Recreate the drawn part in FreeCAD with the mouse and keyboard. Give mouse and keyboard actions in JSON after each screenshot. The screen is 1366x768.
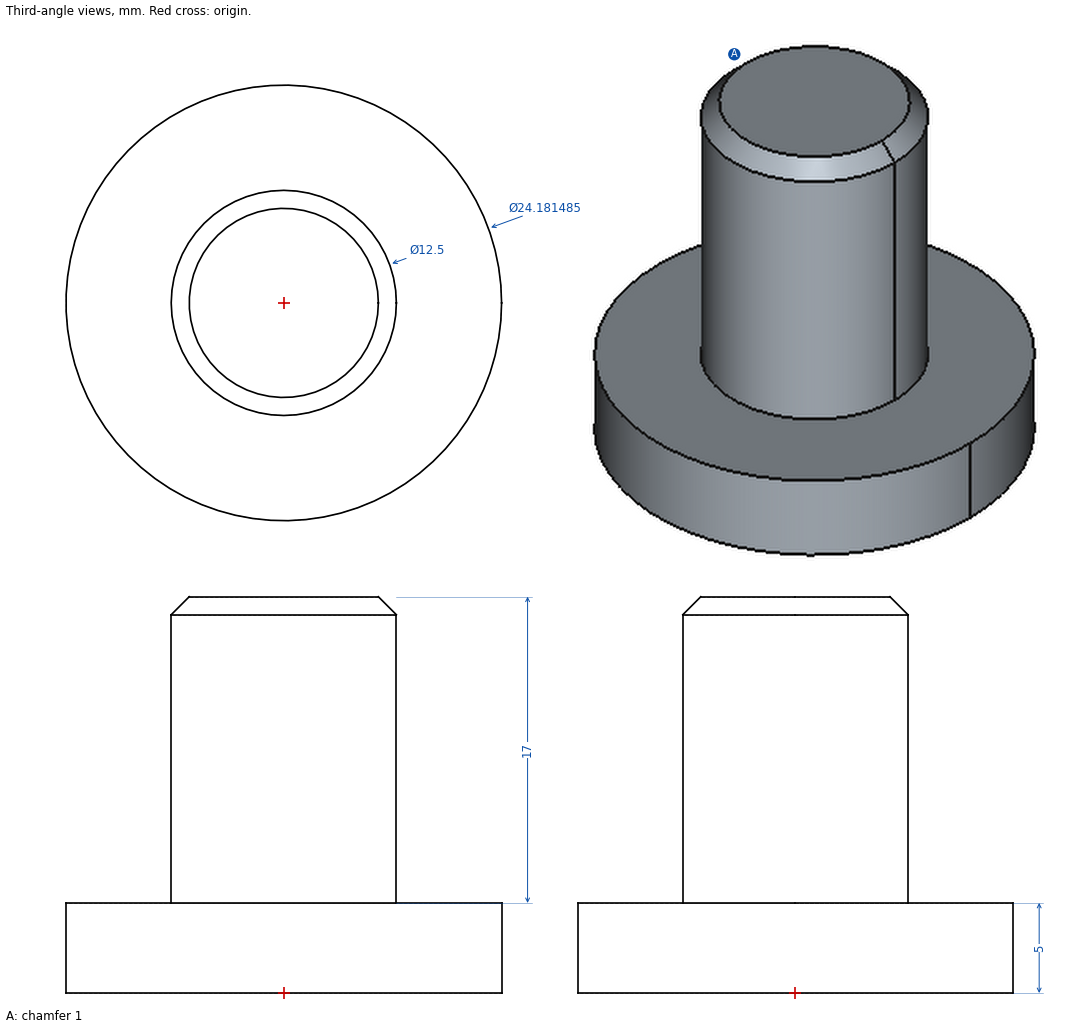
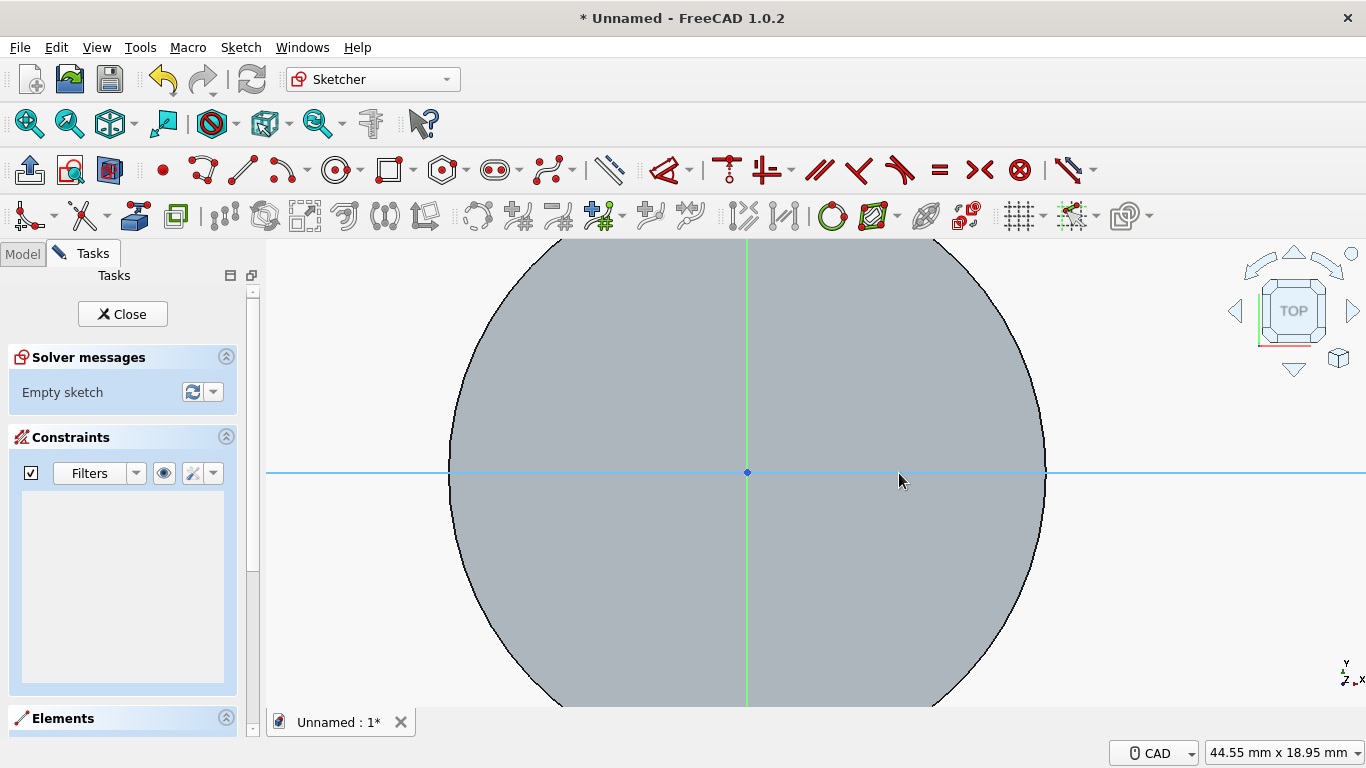
{"action": "left_click", "coordinate": [336, 170]}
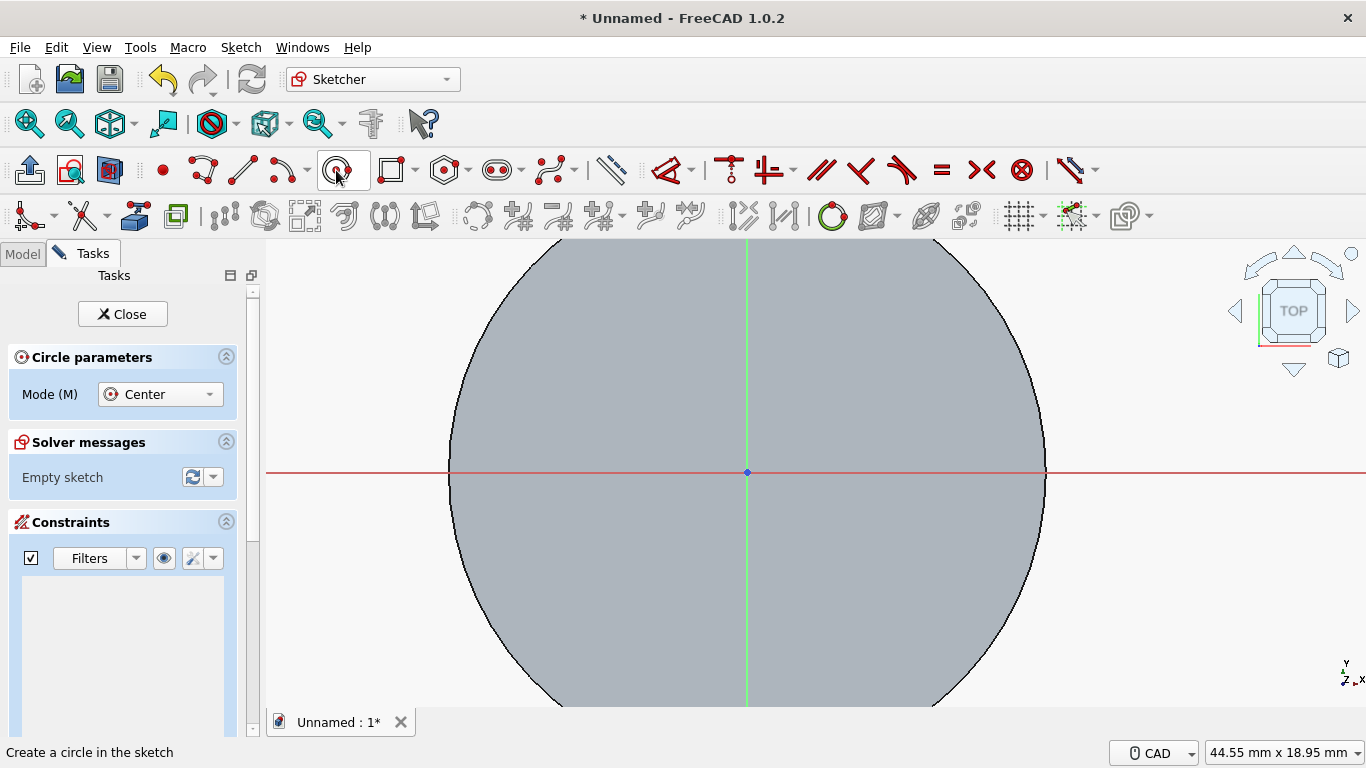
{"action": "left_click", "coordinate": [747, 473]}
{"action": "left_click", "coordinate": [856, 363]}
{"action": "key", "text": "Escape"}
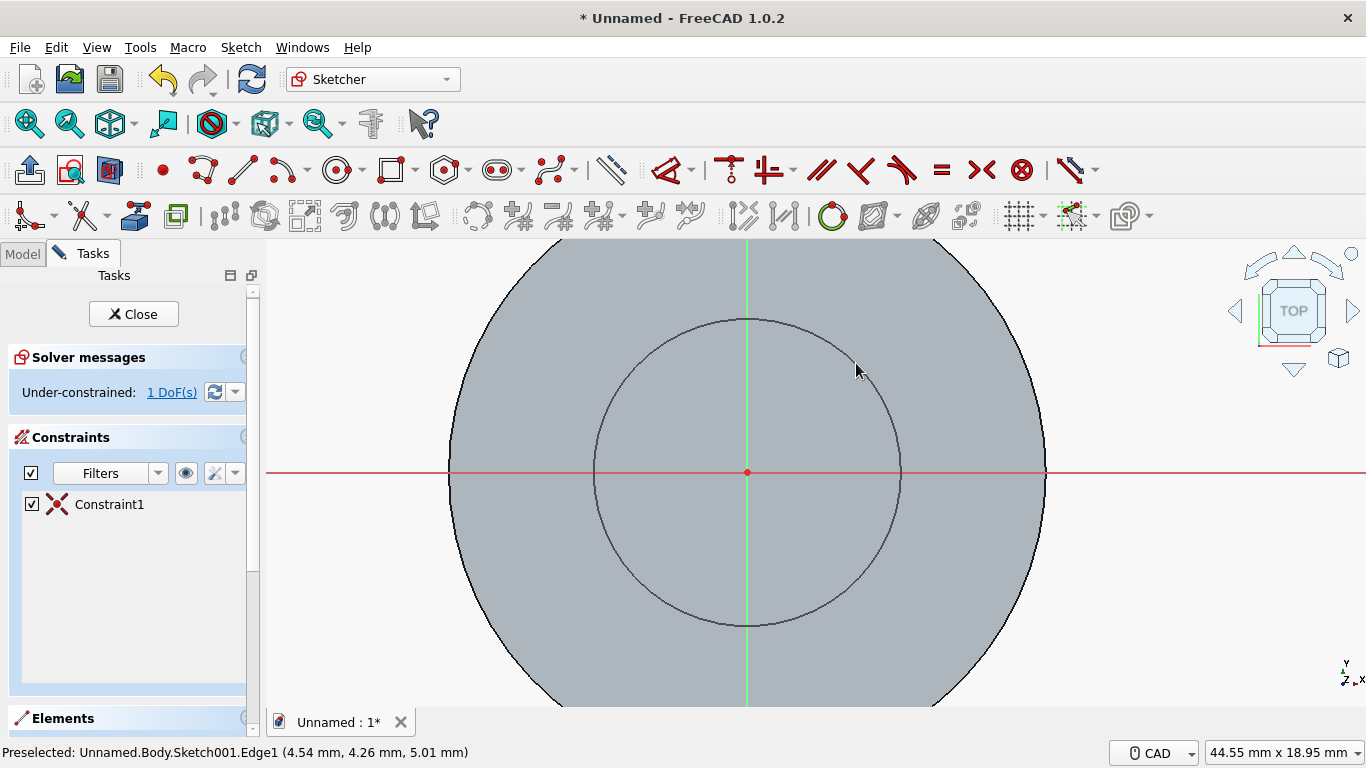
{"action": "left_click", "coordinate": [666, 170]}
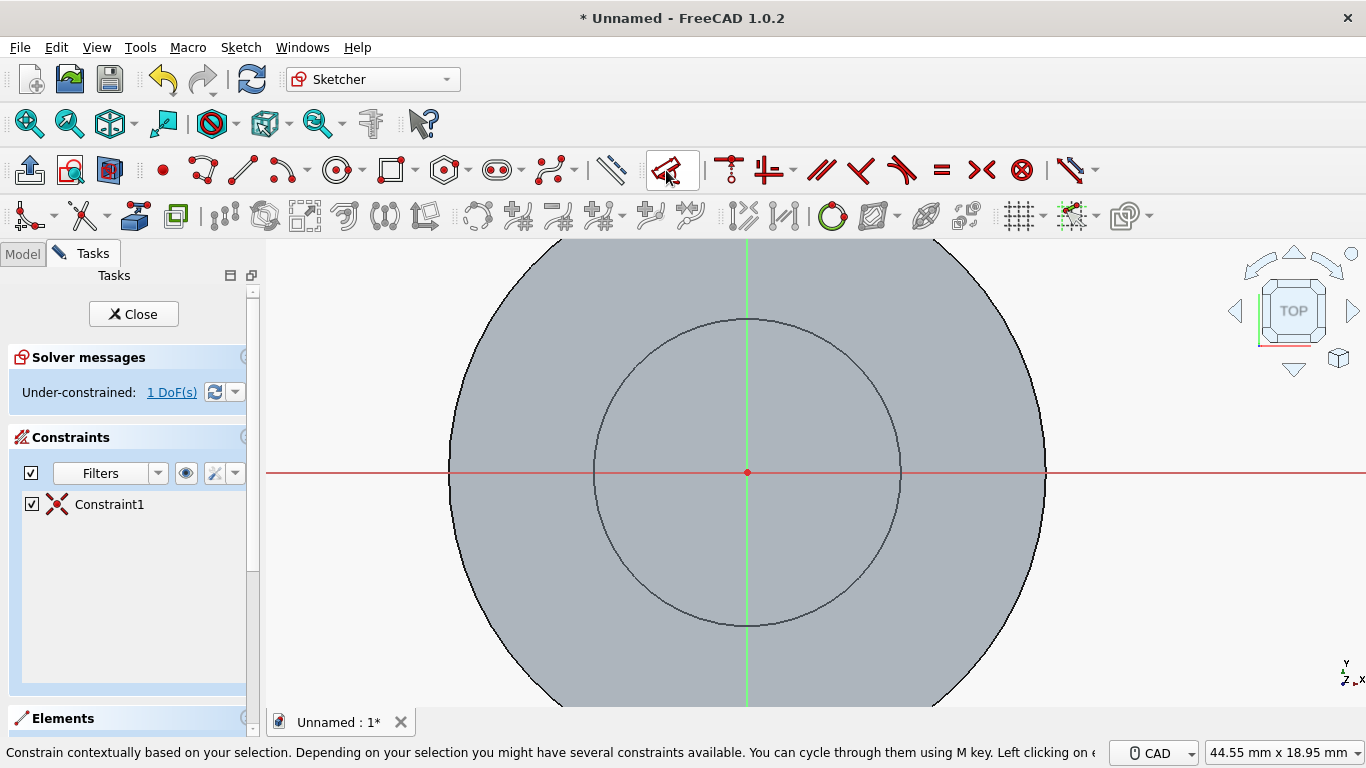
{"action": "left_click", "coordinate": [856, 364]}
{"action": "left_click", "coordinate": [879, 341]}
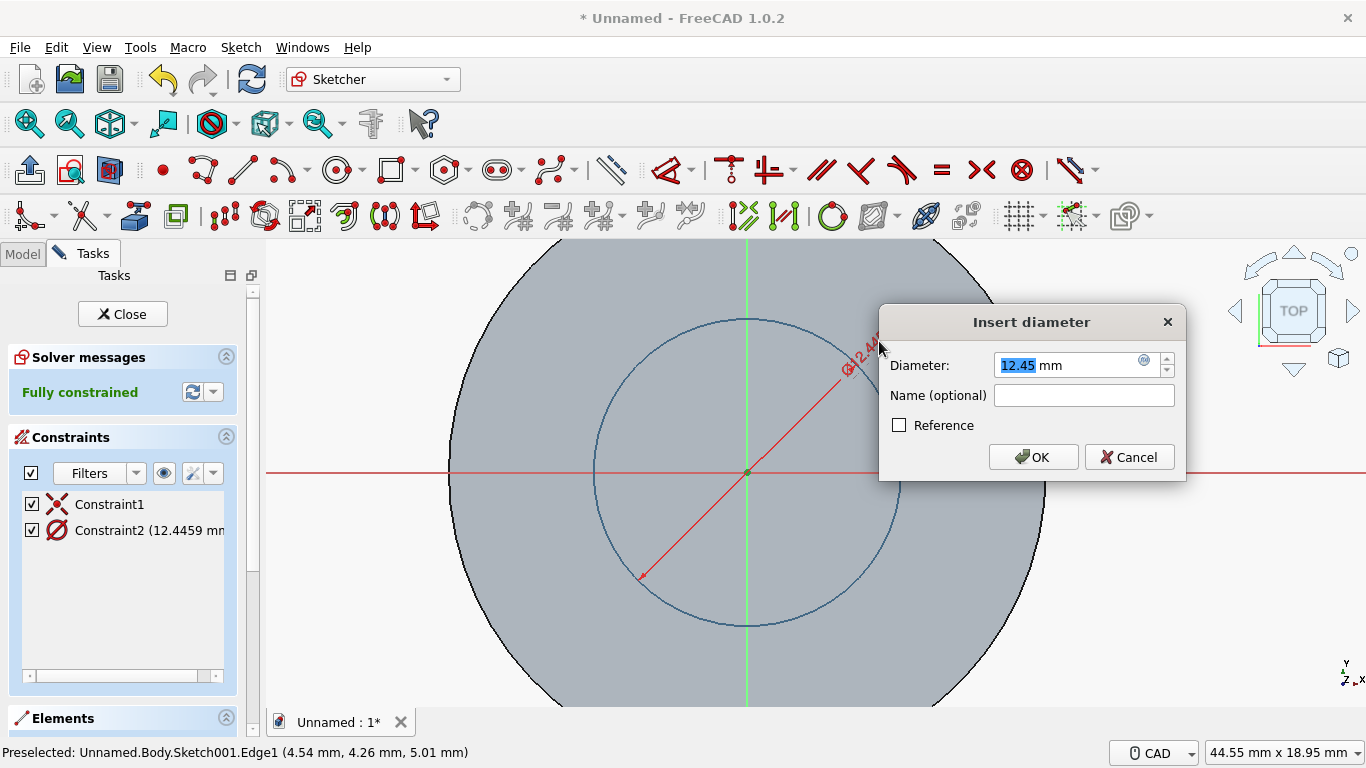
{"action": "type", "text": "12.5"}
{"action": "key", "text": "Return"}
{"action": "key", "text": "Escape"}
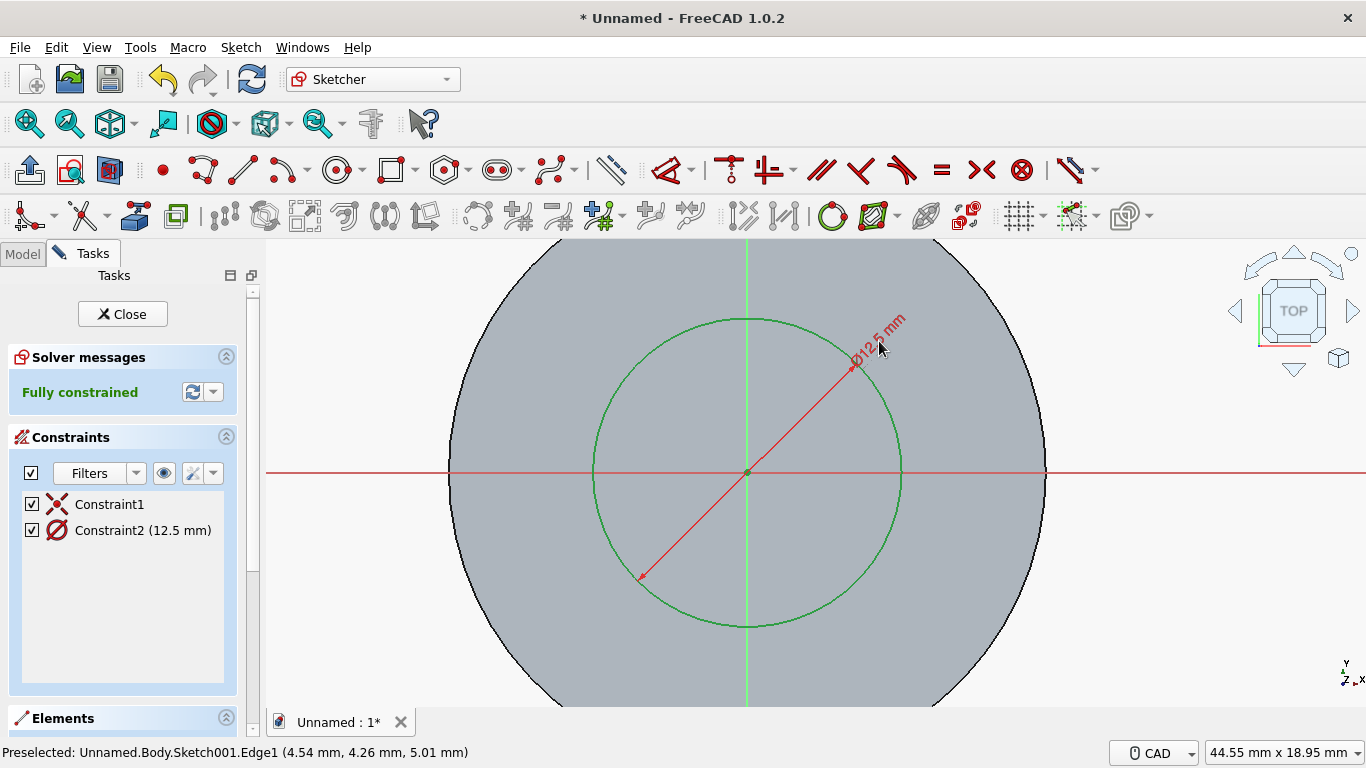
{"action": "left_click", "coordinate": [123, 314]}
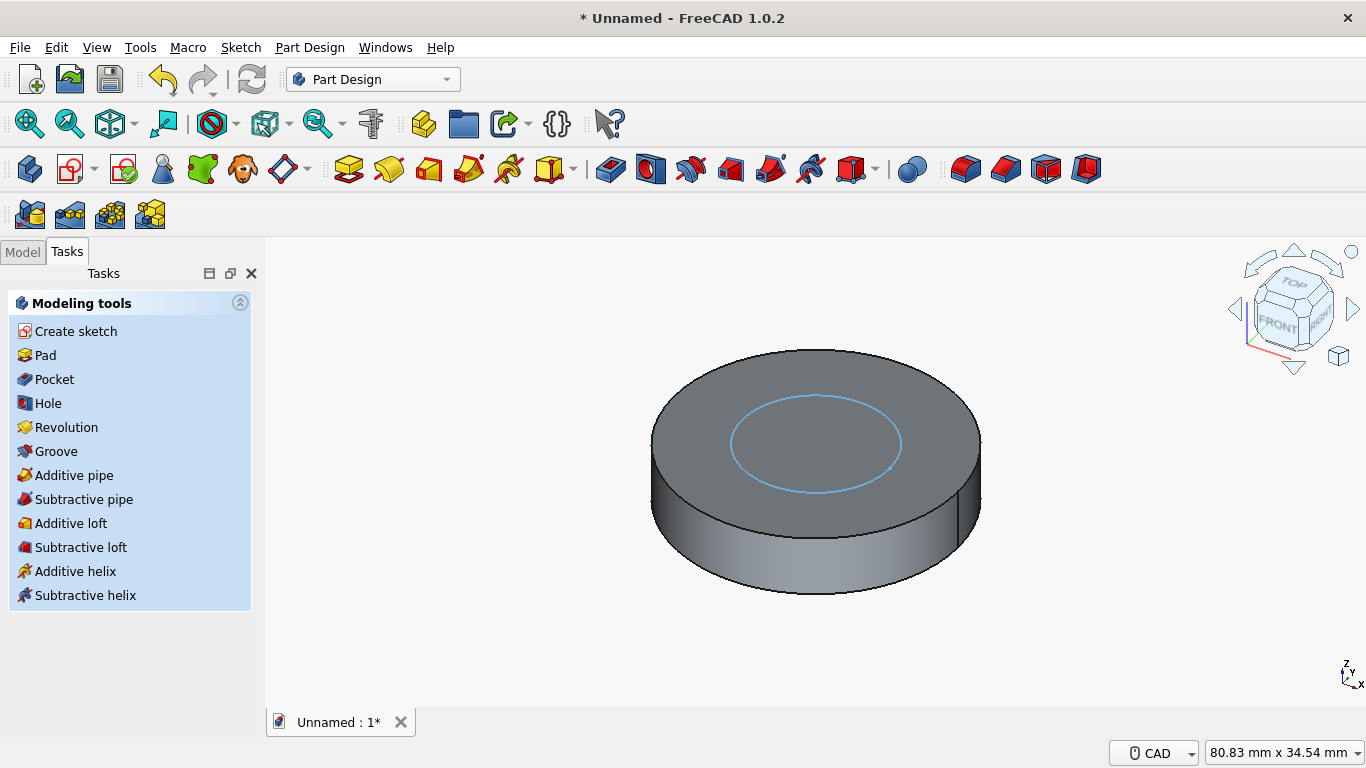
{"action": "left_click", "coordinate": [350, 170]}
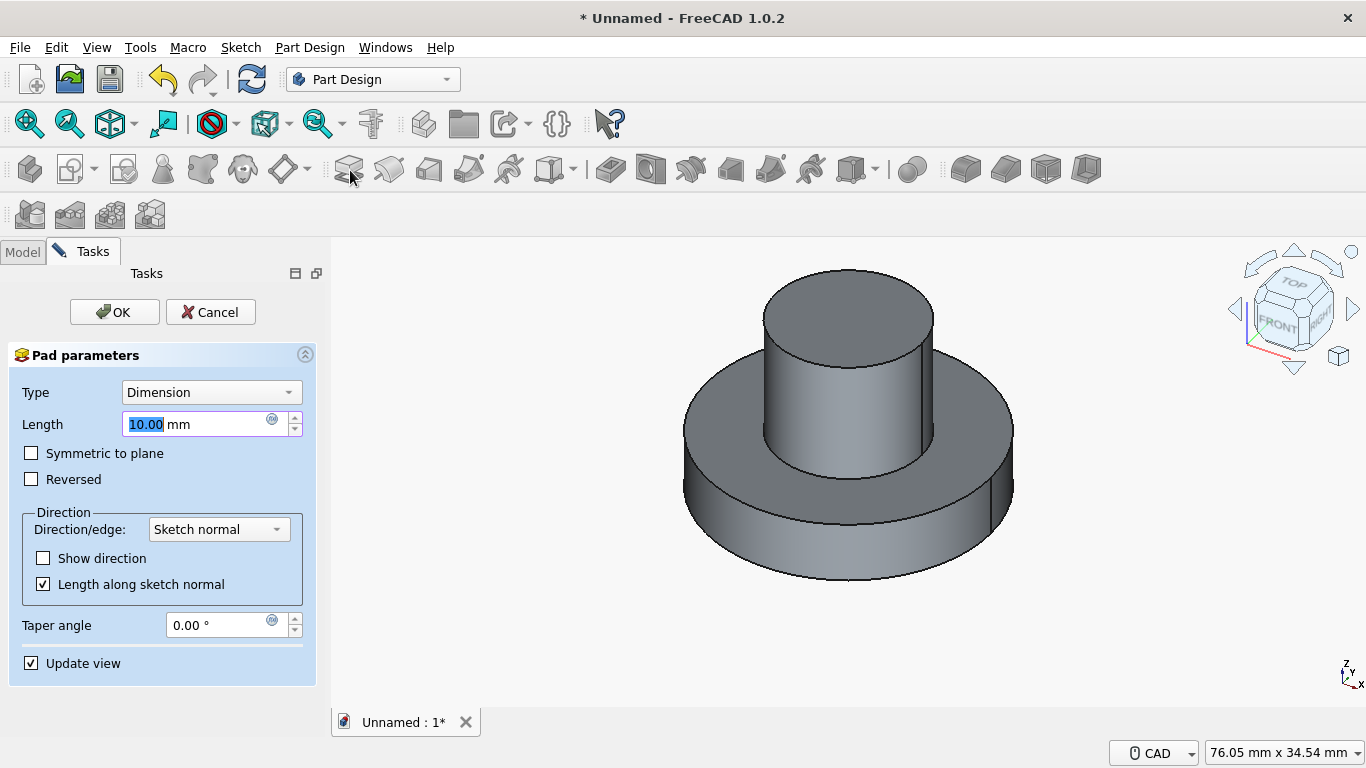
{"action": "type", "text": "17"}
{"action": "key", "text": "Tab"}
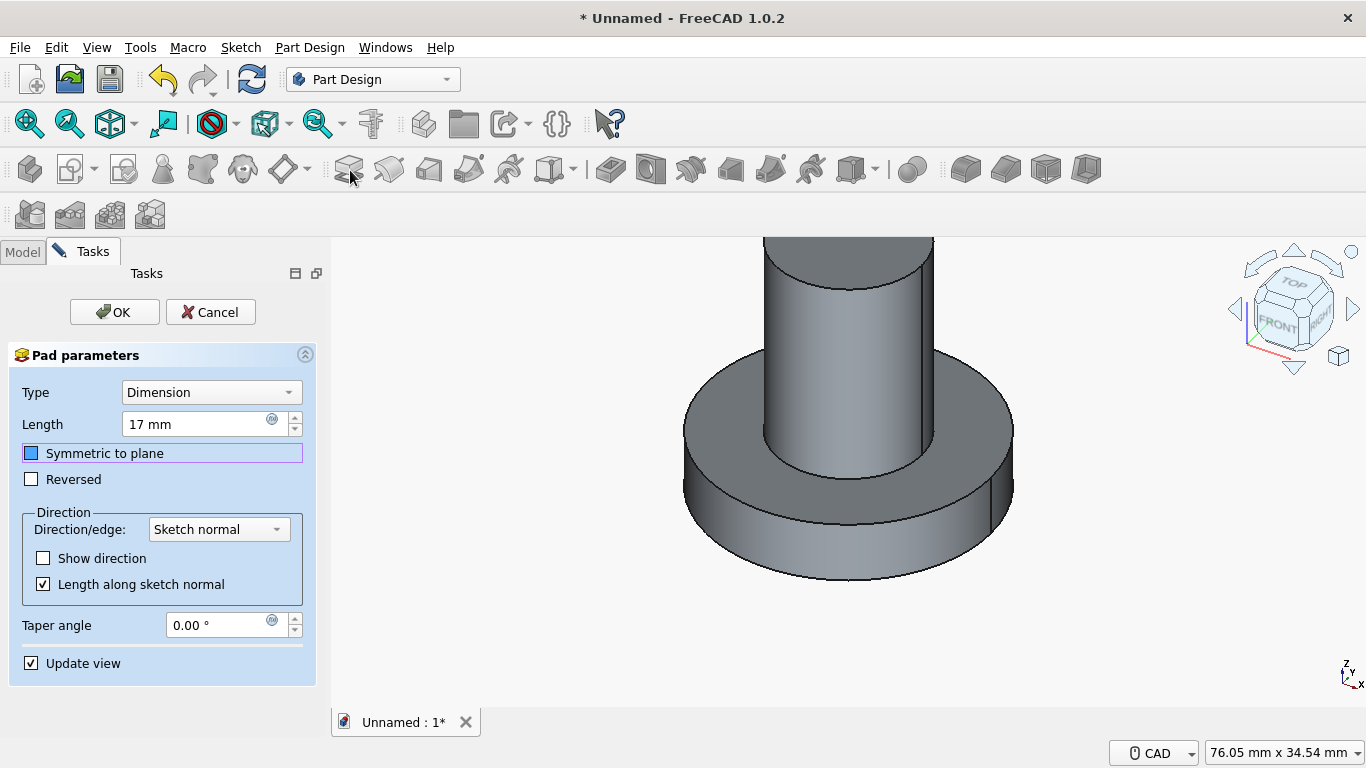
{"action": "left_click", "coordinate": [115, 312]}